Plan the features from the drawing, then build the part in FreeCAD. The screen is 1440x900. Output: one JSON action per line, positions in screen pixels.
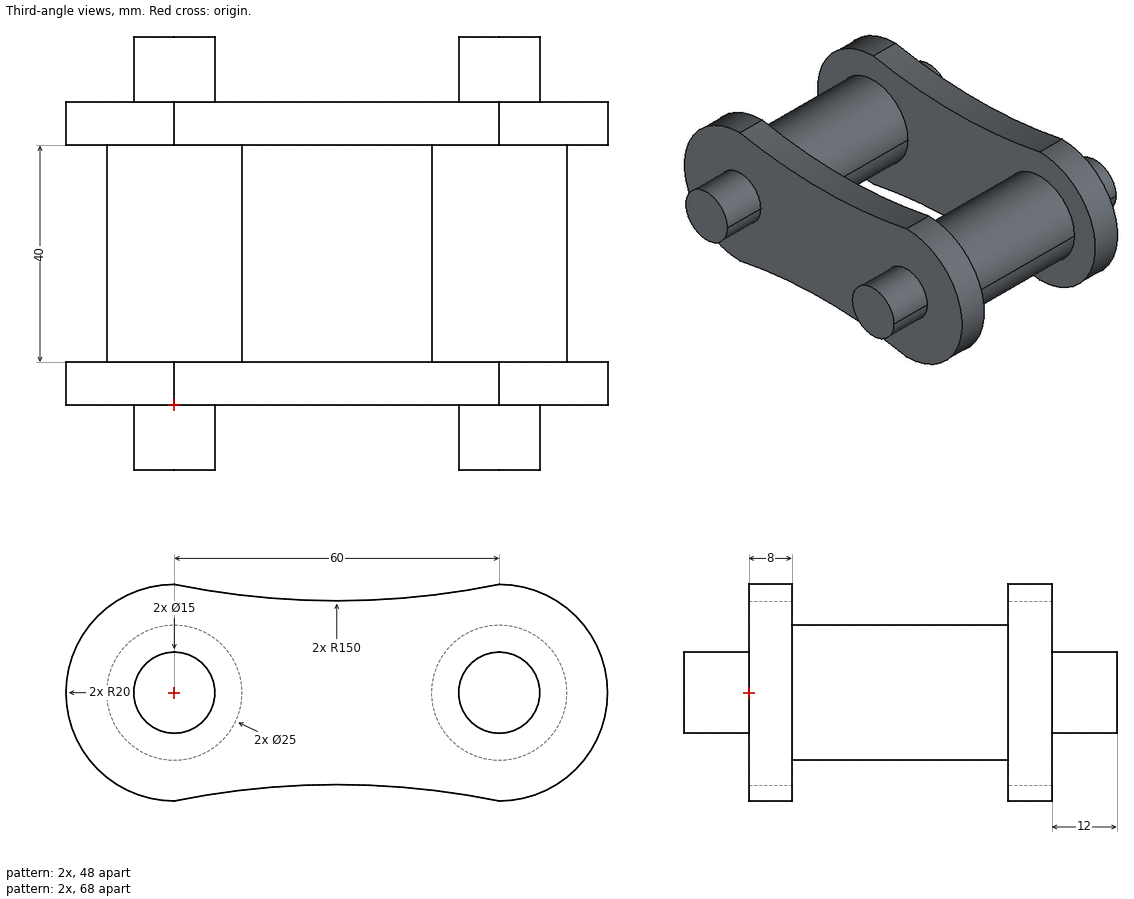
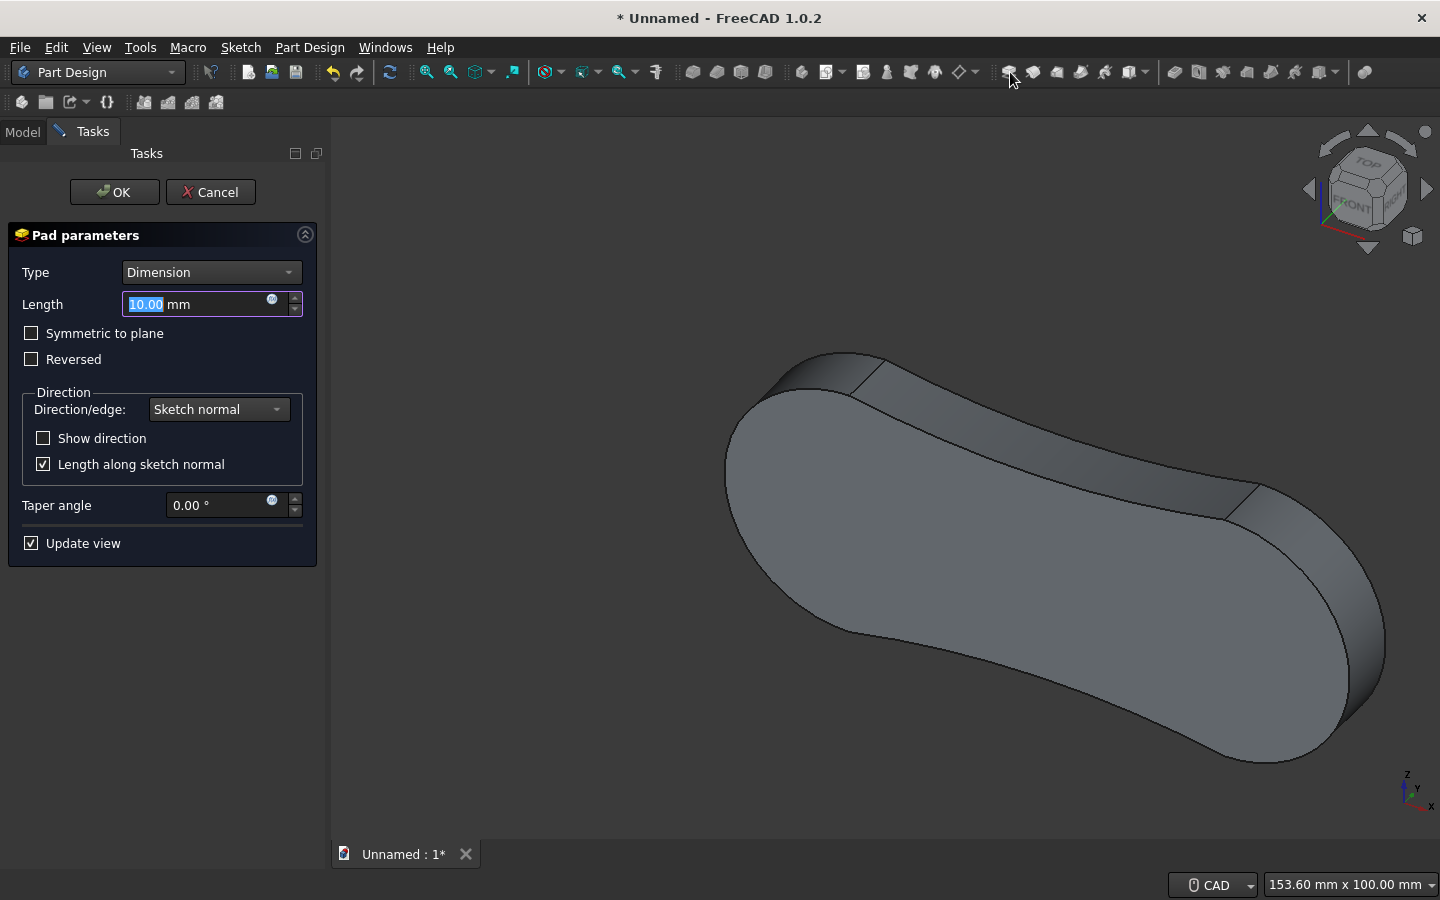
{"action": "type", "text": "8"}
{"action": "key", "text": "Tab"}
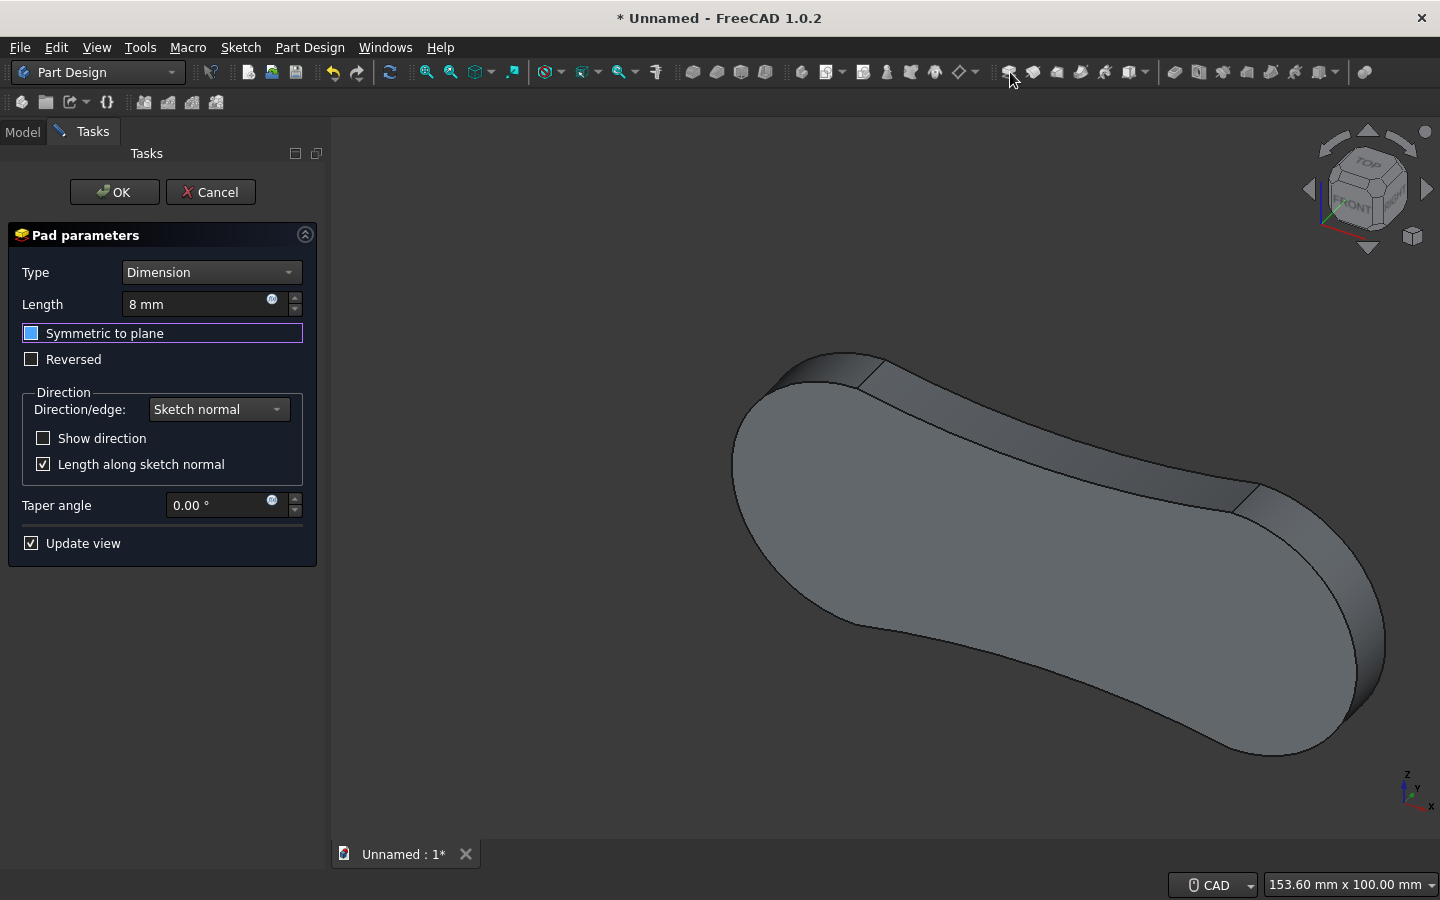
{"action": "left_click", "coordinate": [30, 359]}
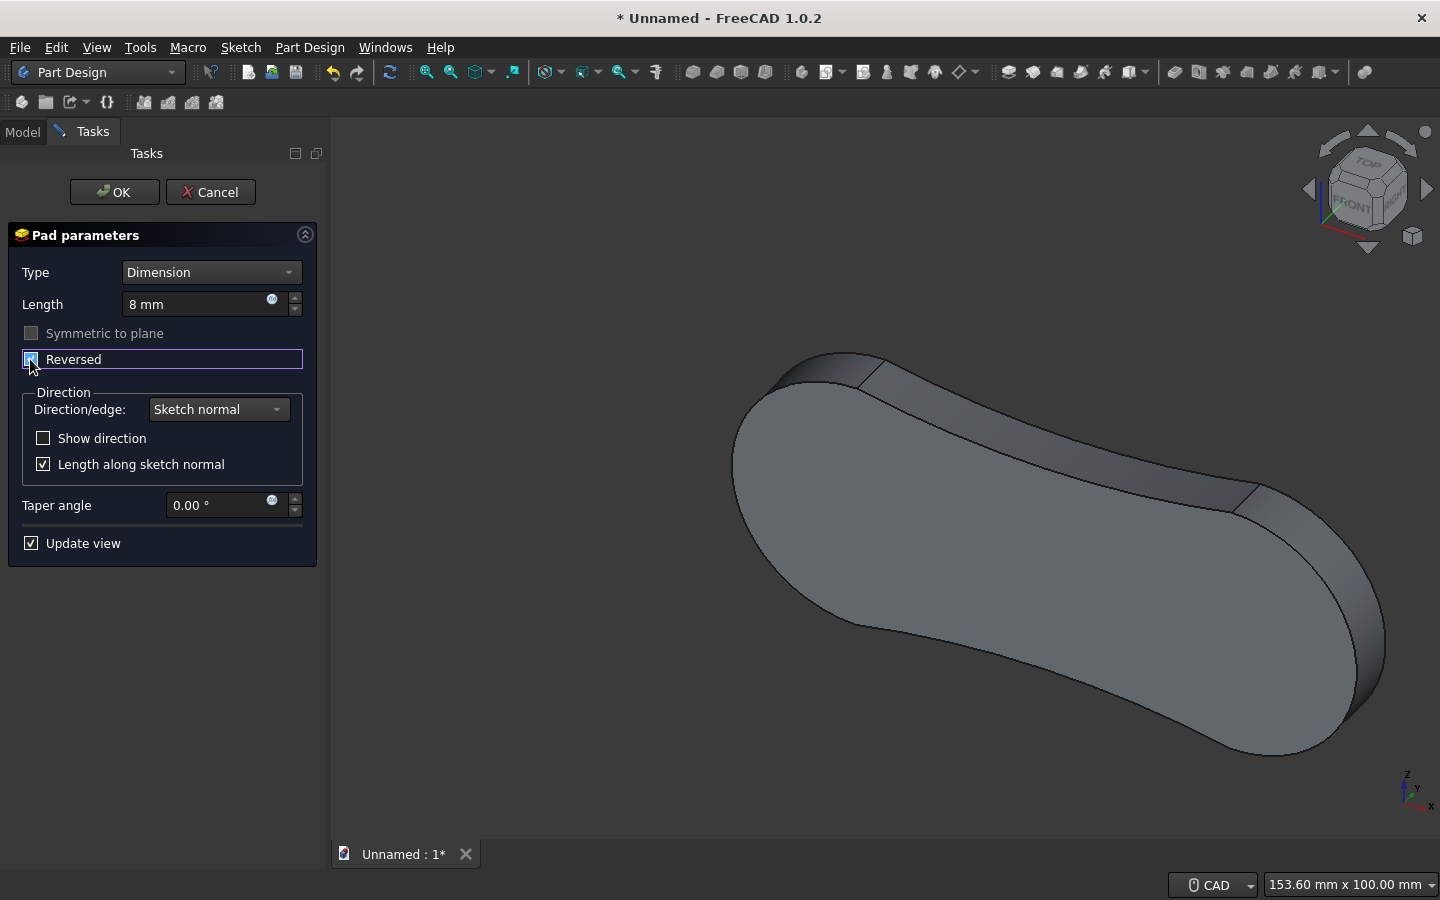
{"action": "left_click", "coordinate": [115, 192]}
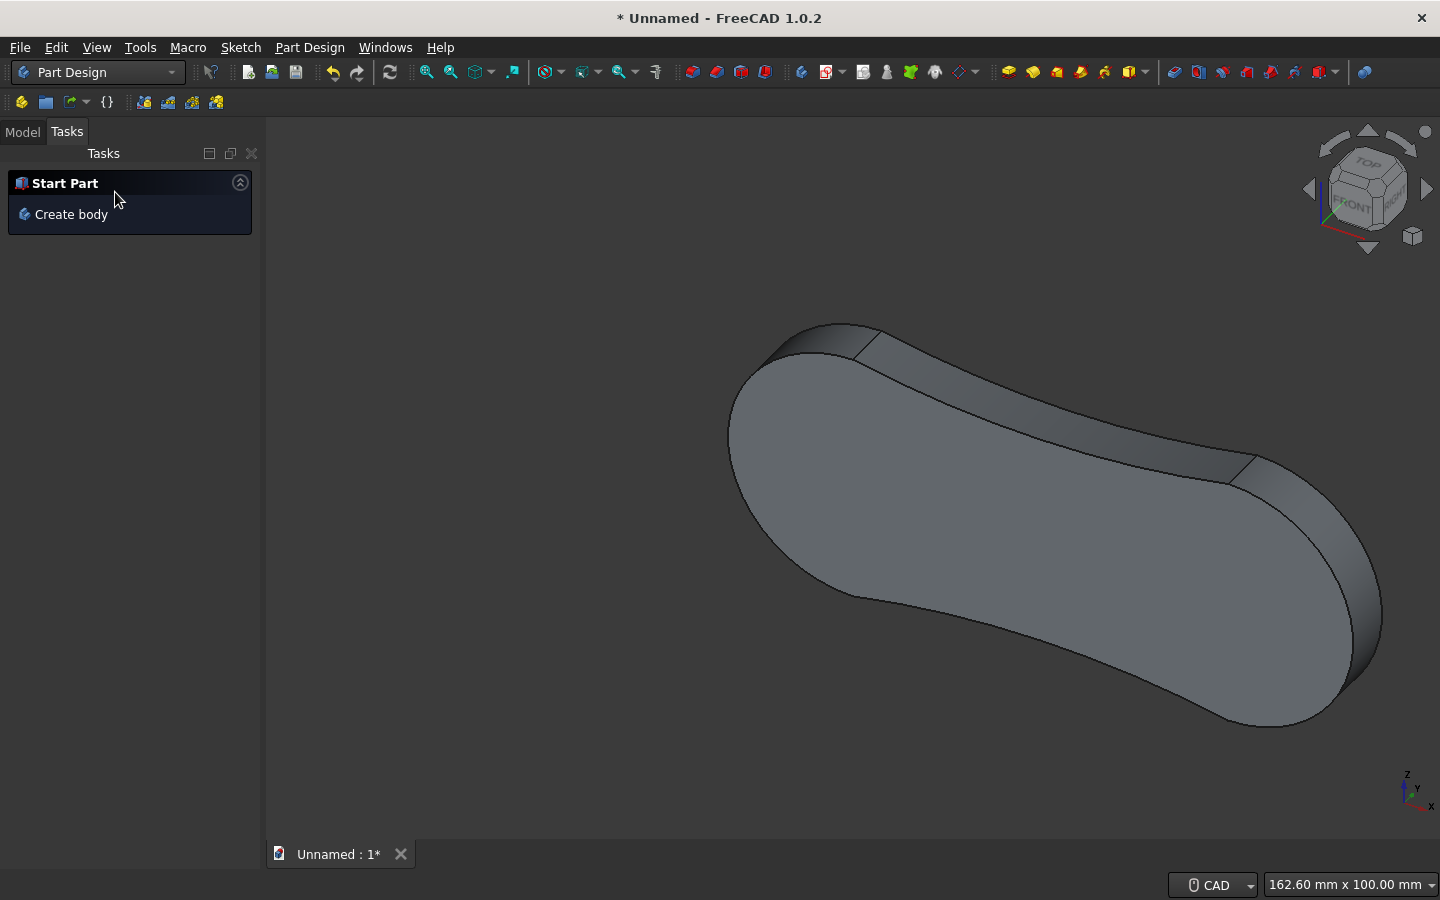
{"action": "key", "text": "4"}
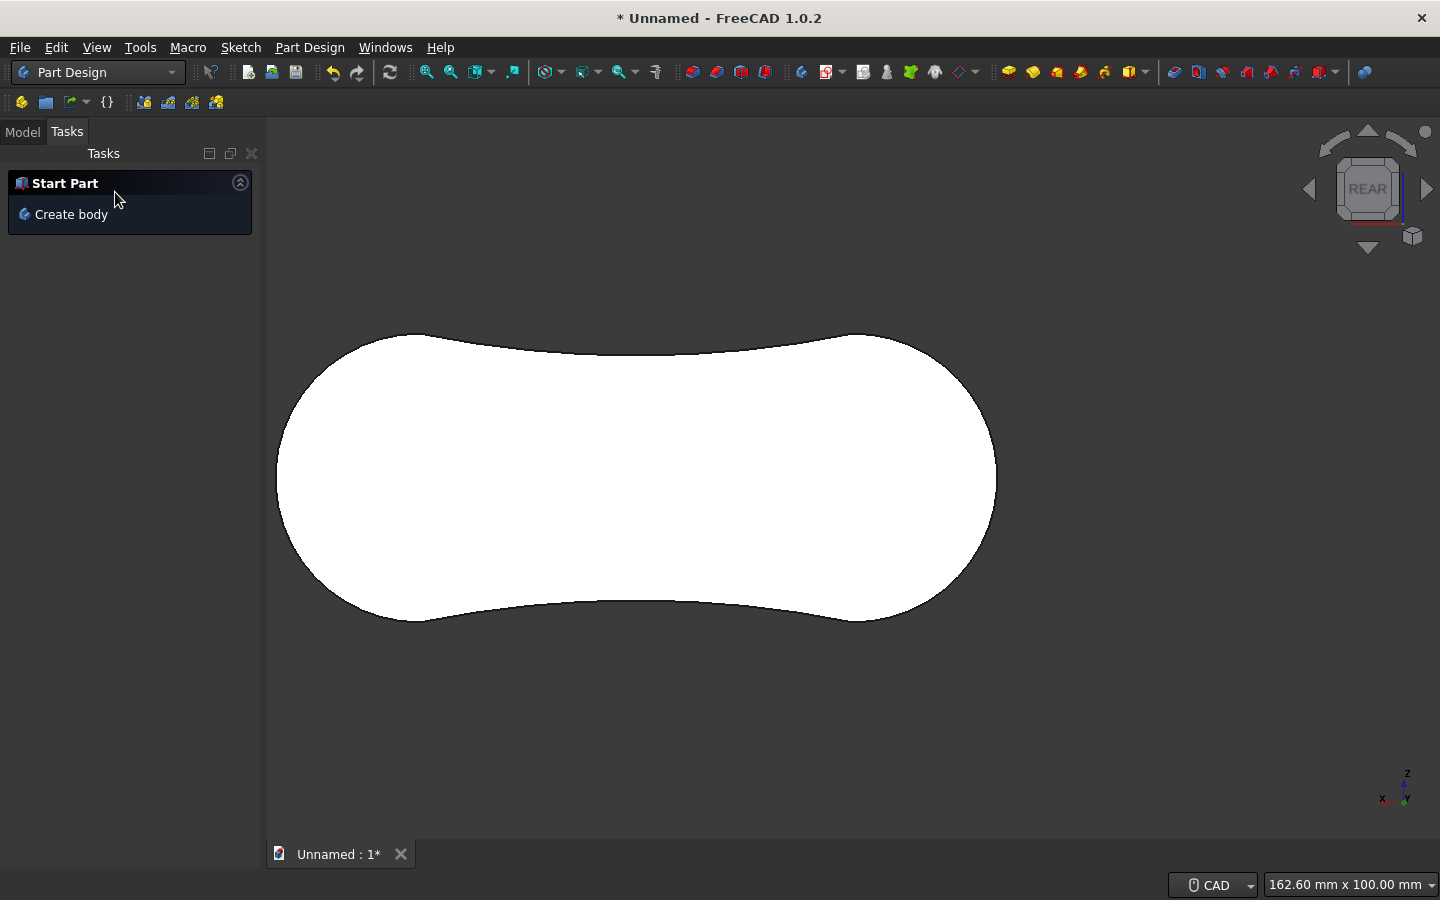
{"action": "left_click", "coordinate": [843, 477]}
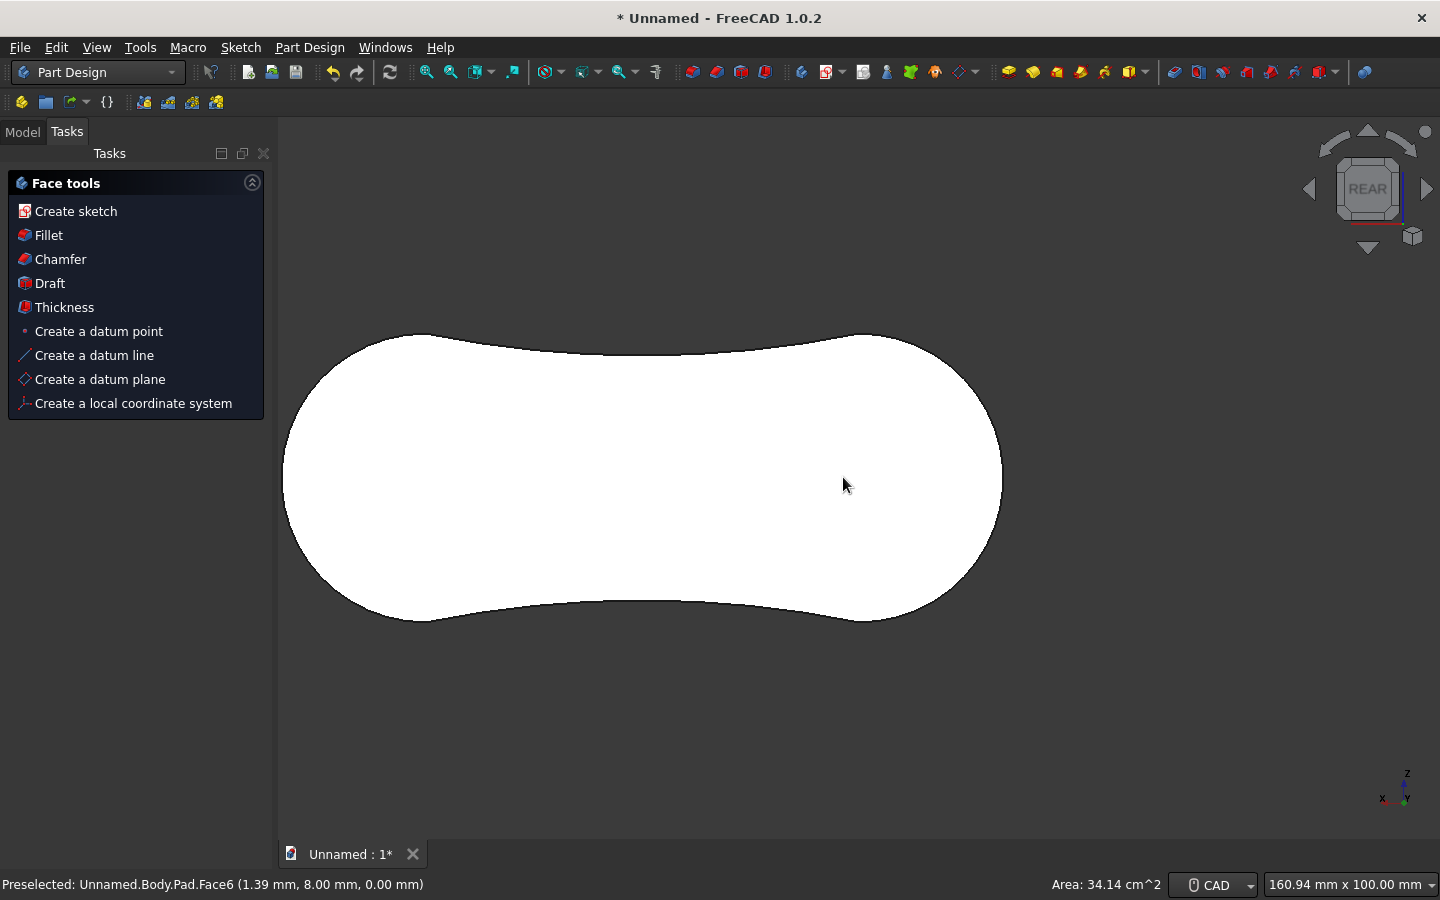
{"action": "left_click", "coordinate": [826, 72]}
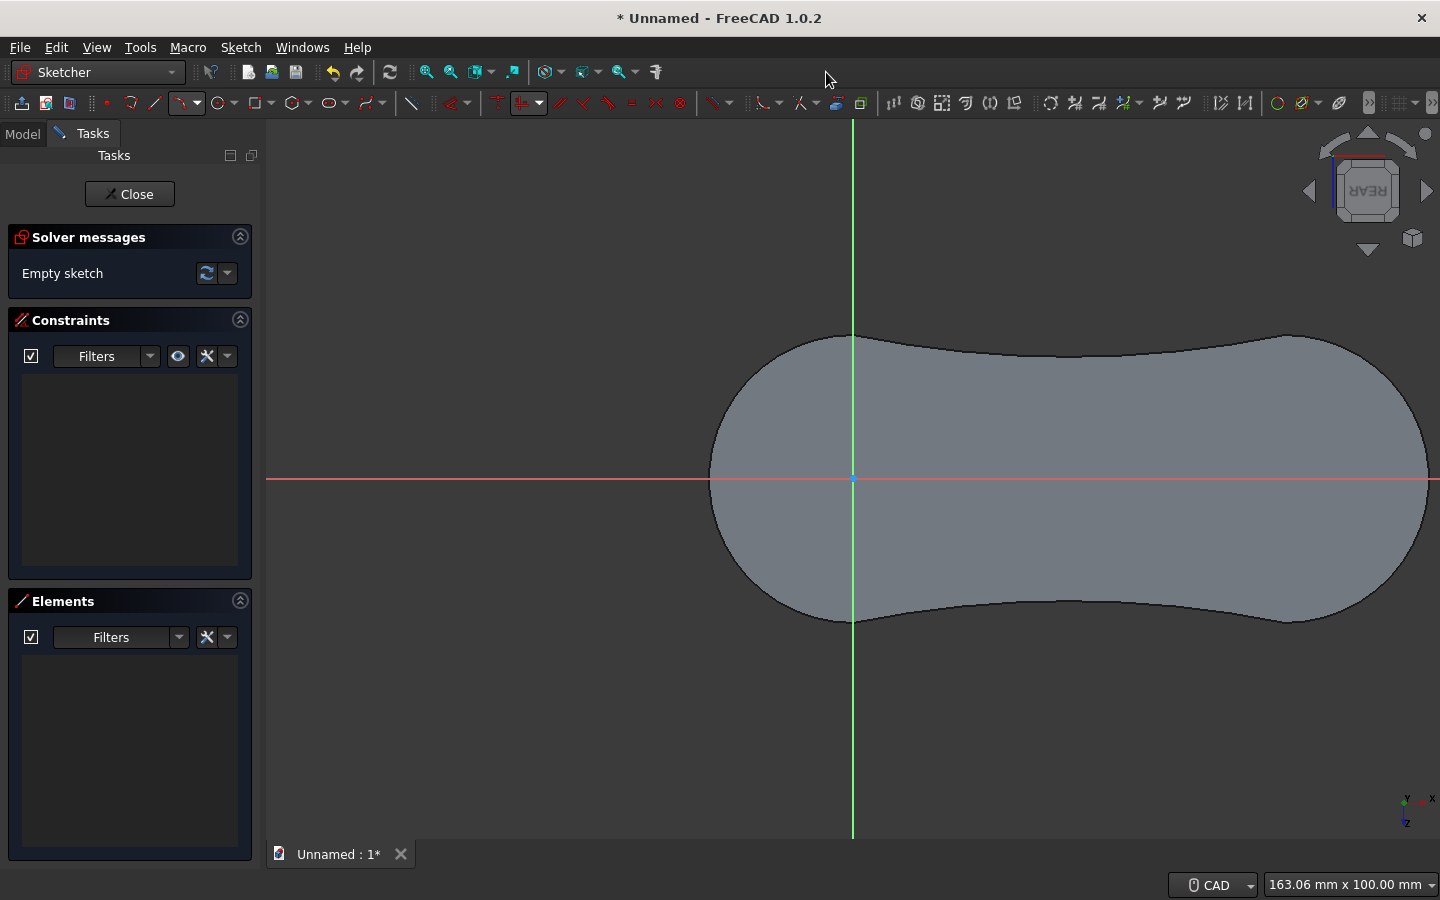
{"action": "scroll", "coordinate": [294, 479], "scroll_direction": "down", "scroll_amount": 1}